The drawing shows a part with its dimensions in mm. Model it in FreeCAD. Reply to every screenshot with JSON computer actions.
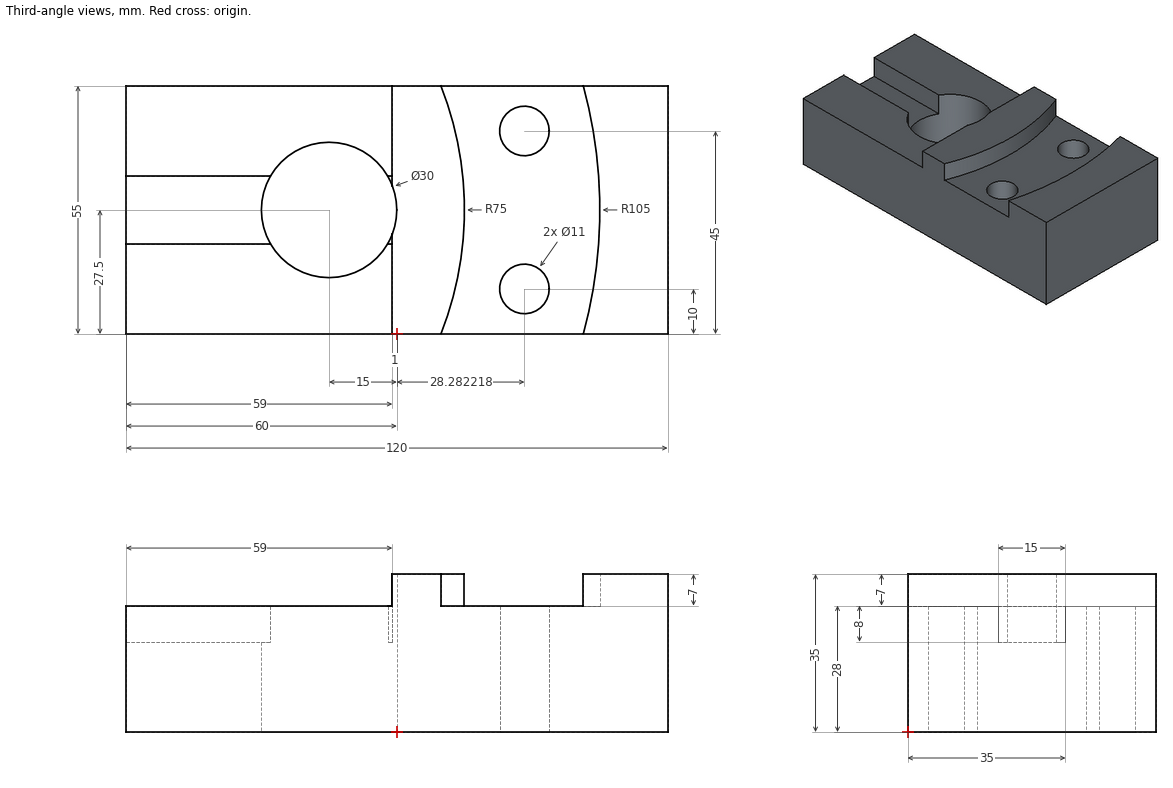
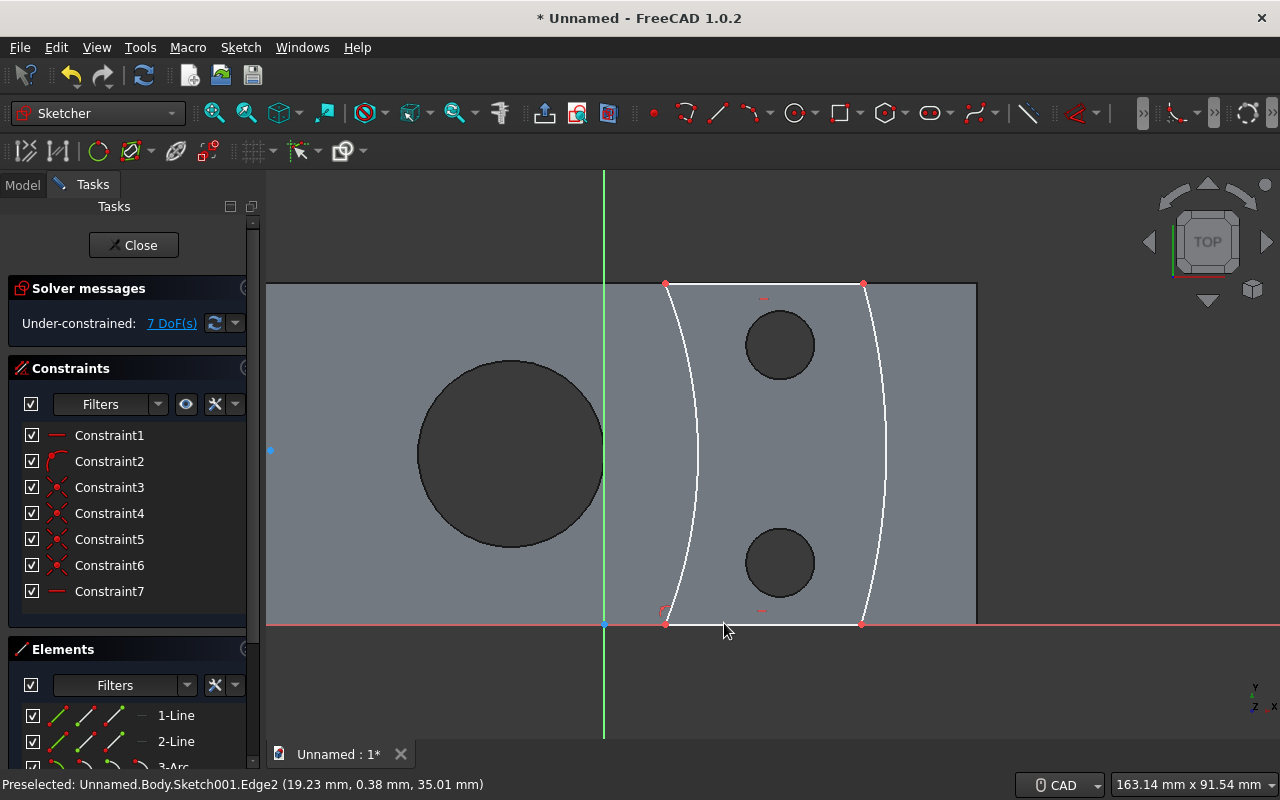
{"action": "left_click", "coordinate": [693, 524]}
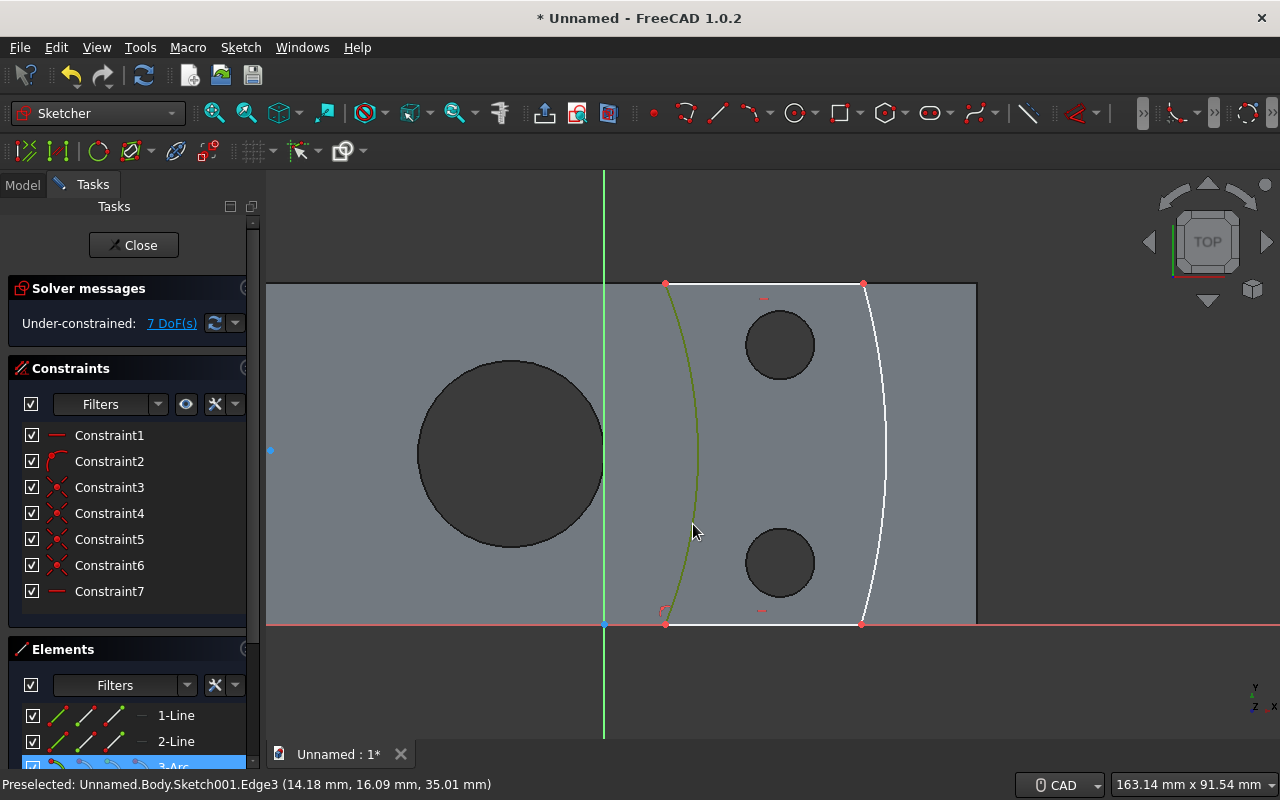
{"action": "left_click", "coordinate": [882, 524]}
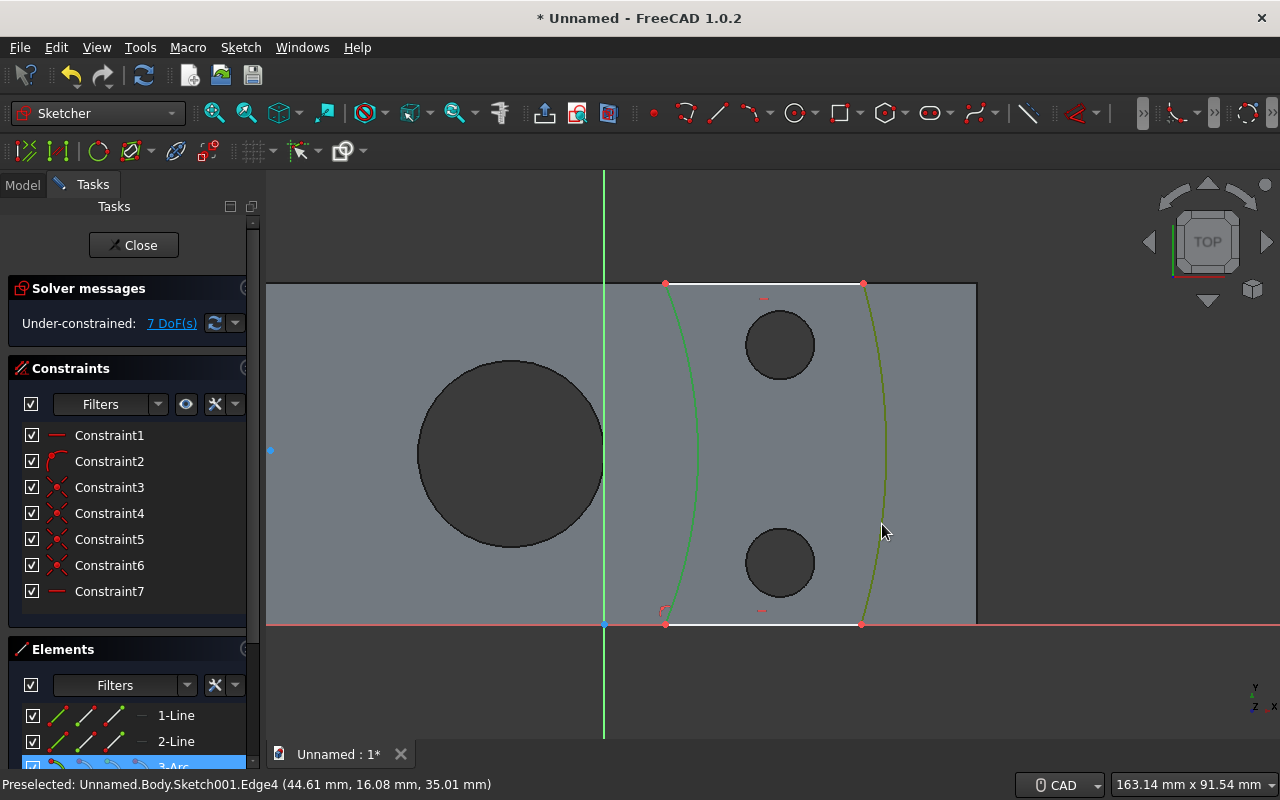
{"action": "key", "text": "c"}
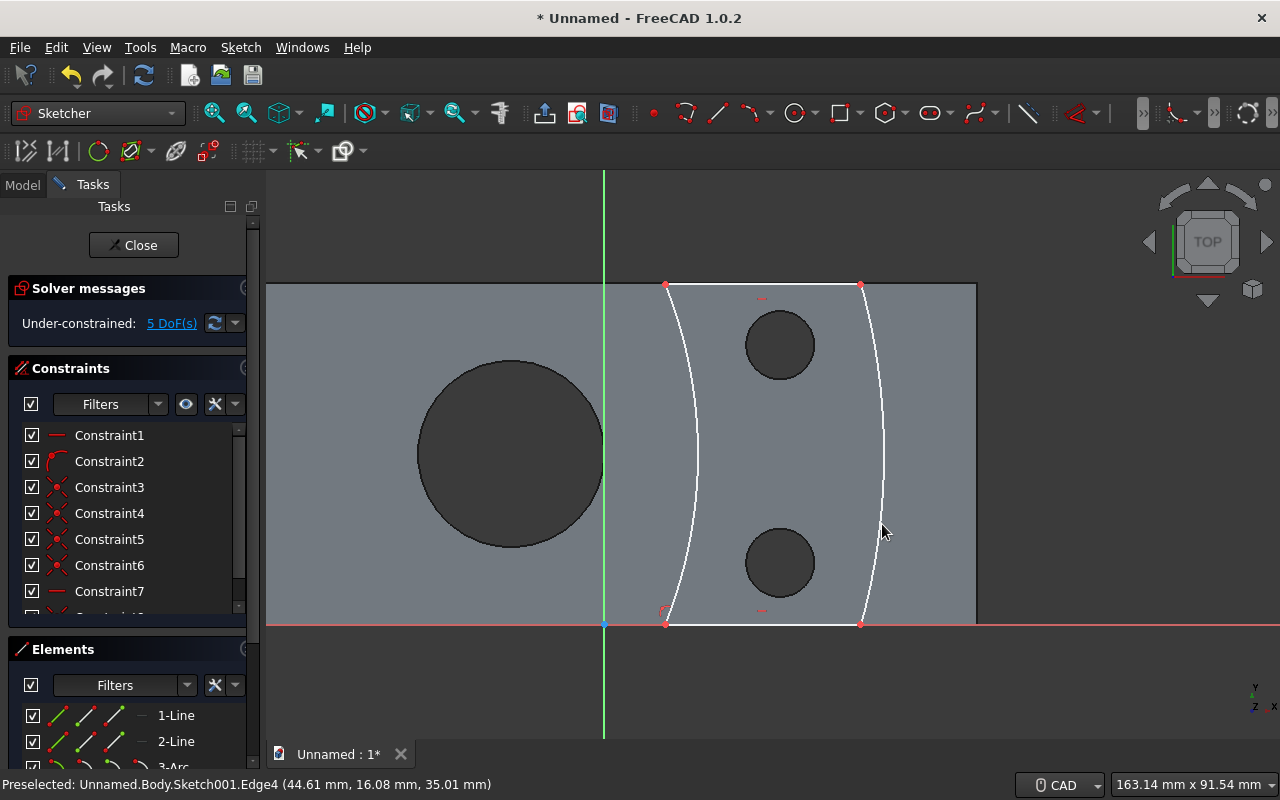
{"action": "key", "text": "d"}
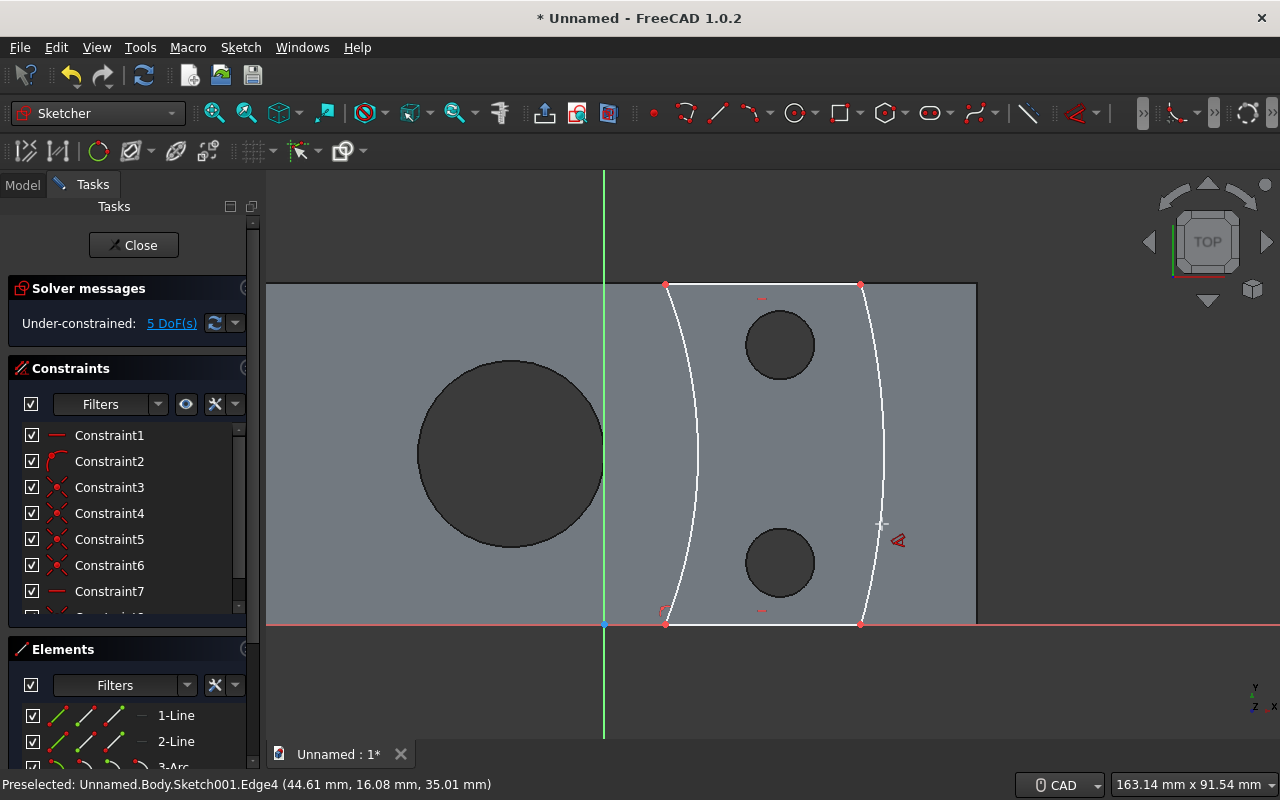
{"action": "left_click", "coordinate": [693, 524]}
{"action": "left_click", "coordinate": [725, 529]}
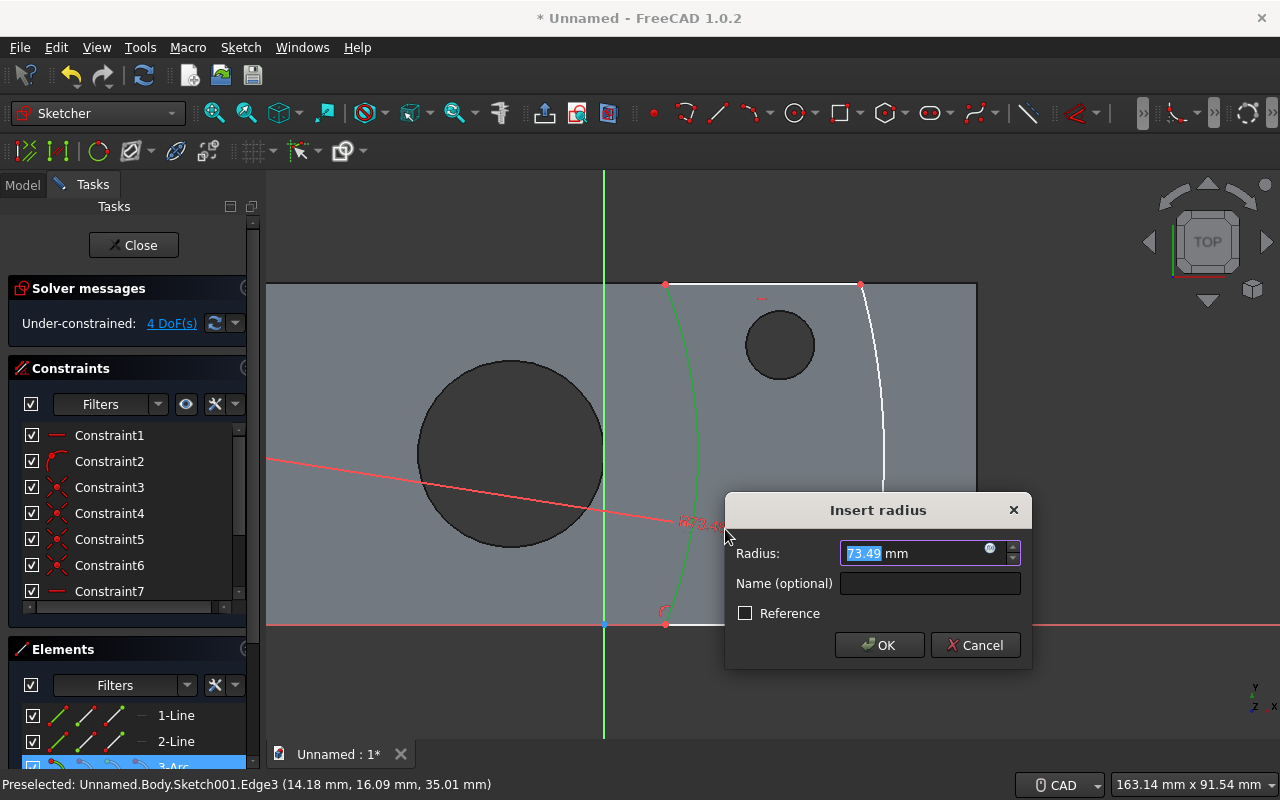
{"action": "type", "text": "75"}
{"action": "key", "text": "Return"}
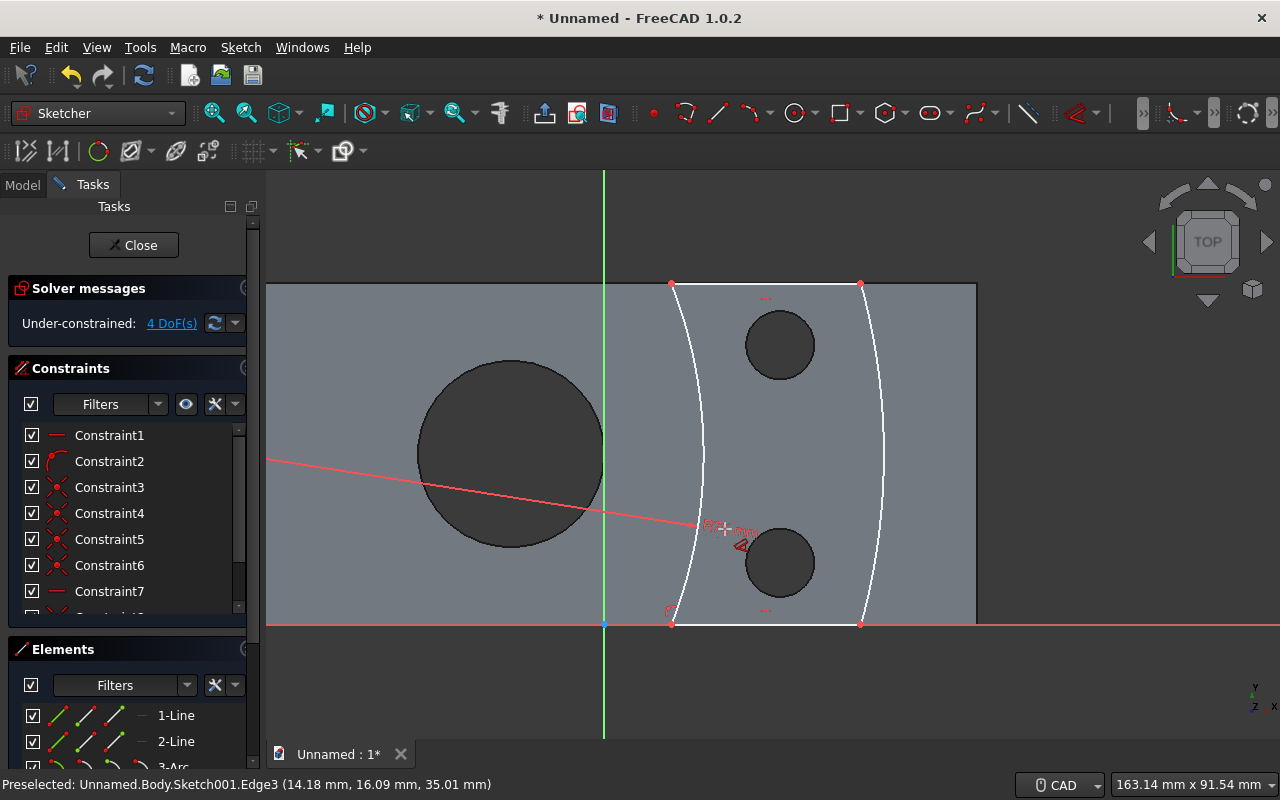
{"action": "left_click", "coordinate": [880, 523]}
{"action": "left_click", "coordinate": [912, 526]}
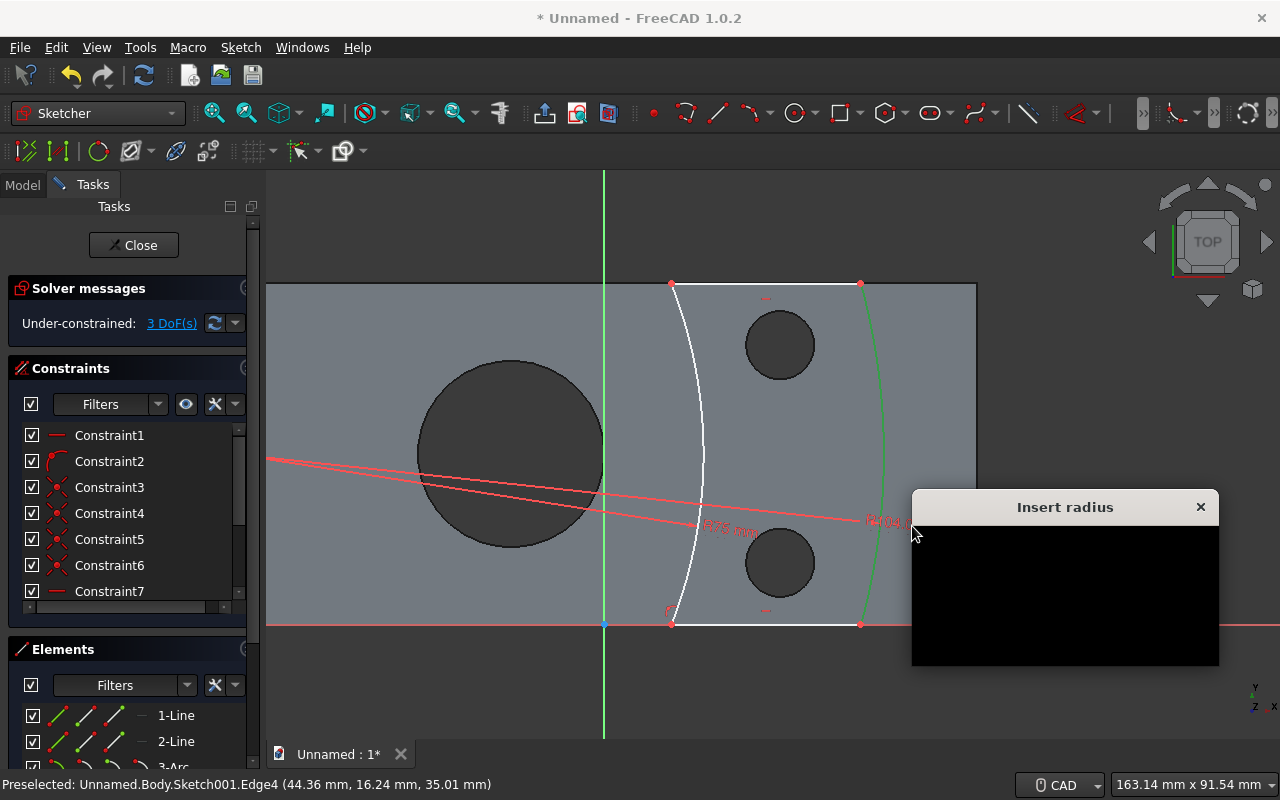
{"action": "type", "text": "105"}
{"action": "key", "text": "Return"}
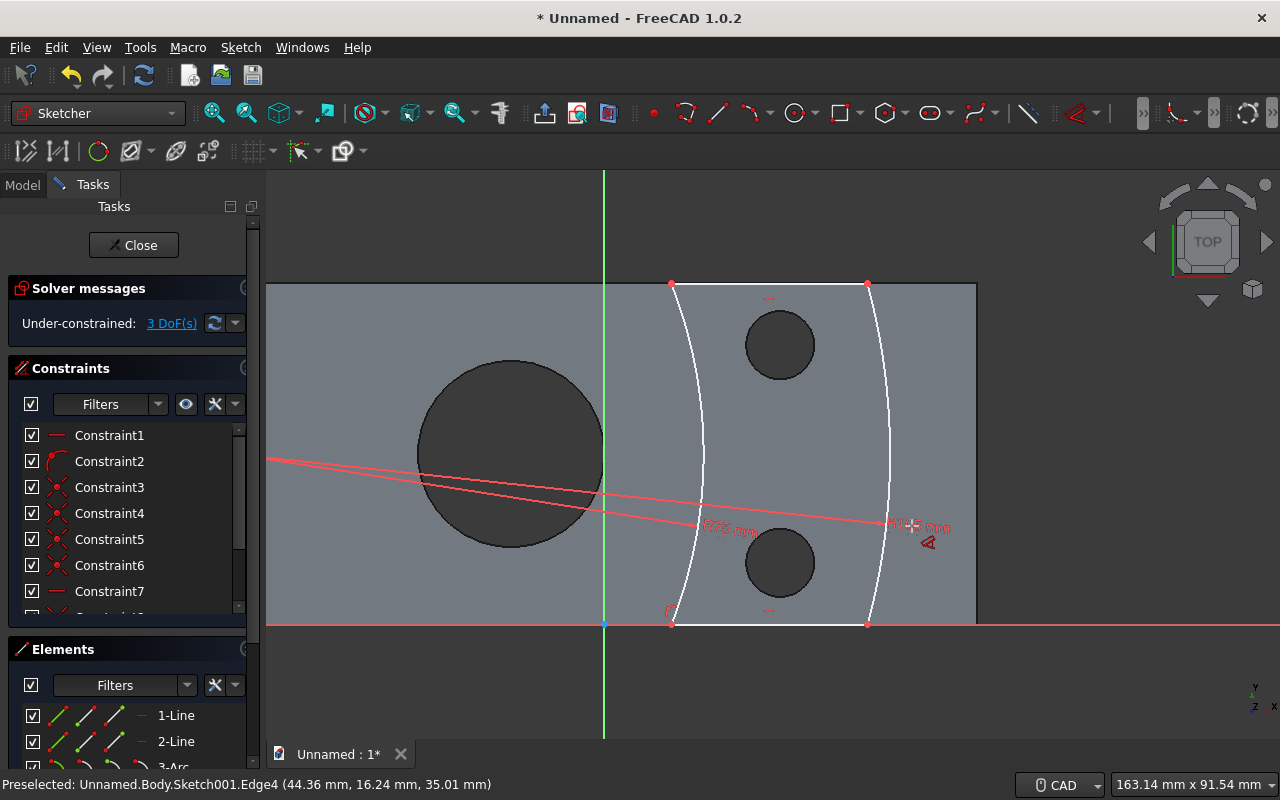
{"action": "left_click", "coordinate": [867, 284]}
{"action": "left_click", "coordinate": [570, 454]}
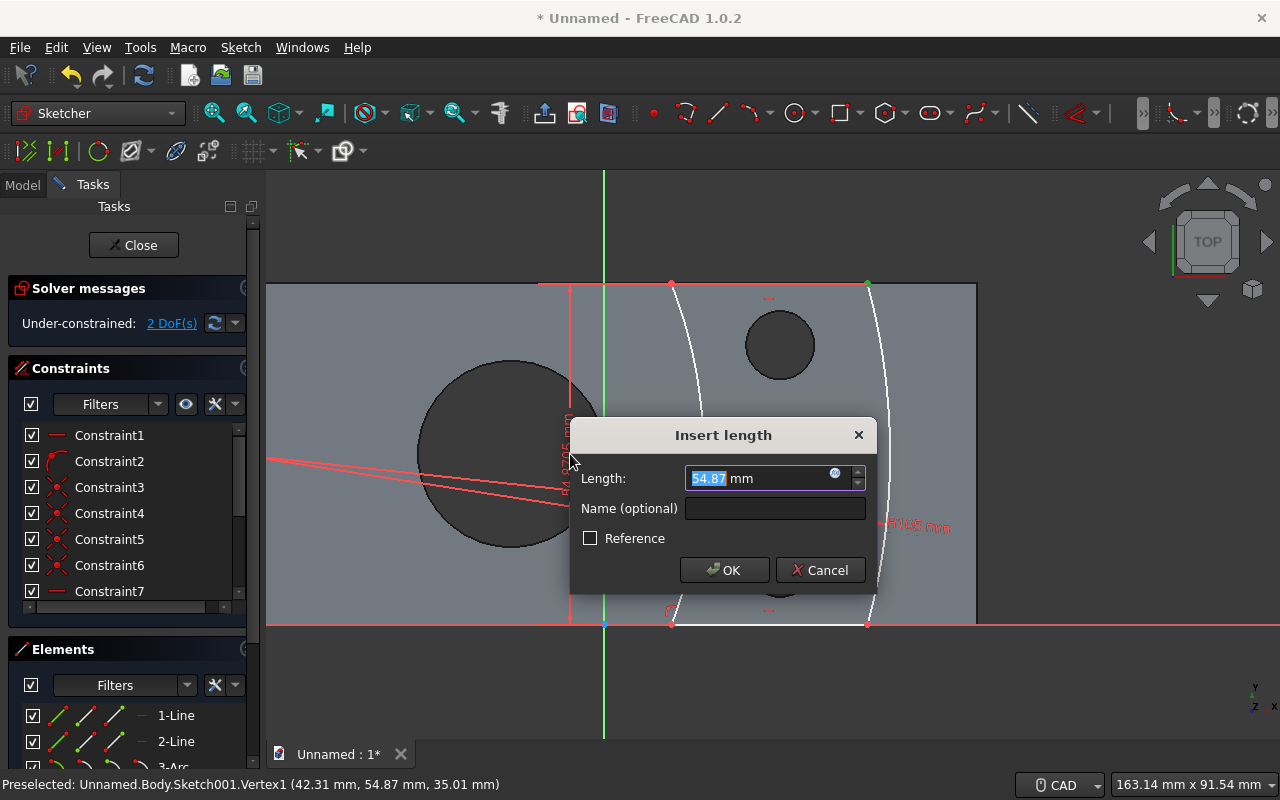
{"action": "type", "text": "55"}
{"action": "key", "text": "Return"}